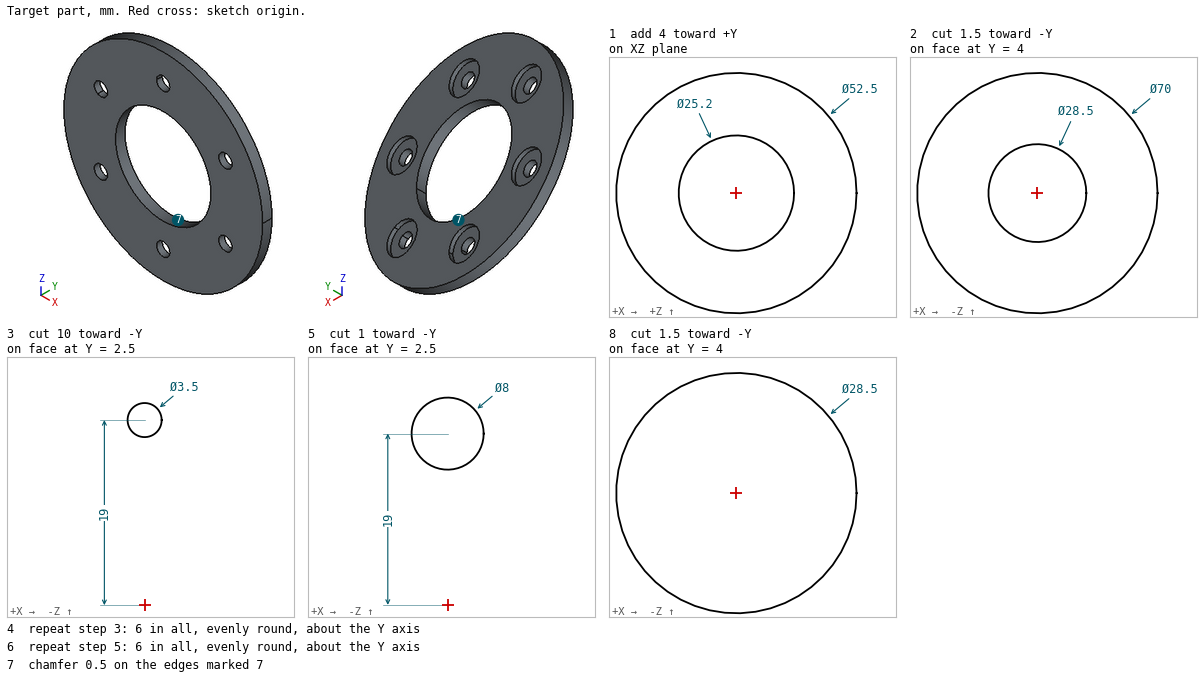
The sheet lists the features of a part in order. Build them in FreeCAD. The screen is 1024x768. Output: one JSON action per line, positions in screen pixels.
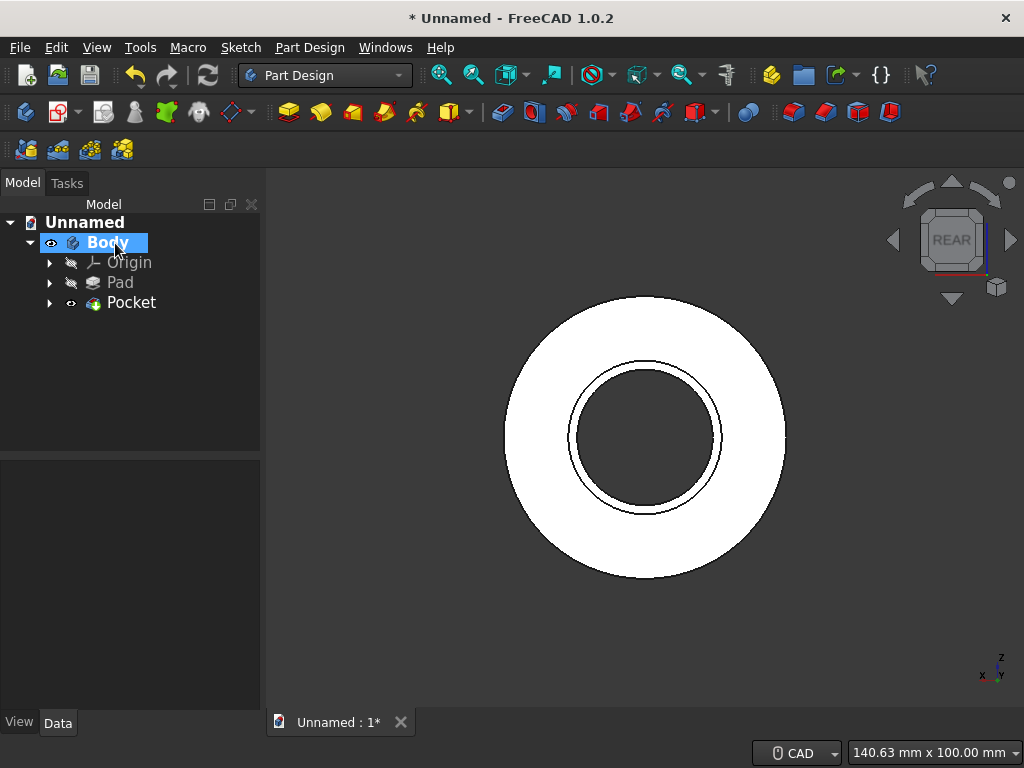
{"action": "left_click", "coordinate": [564, 356]}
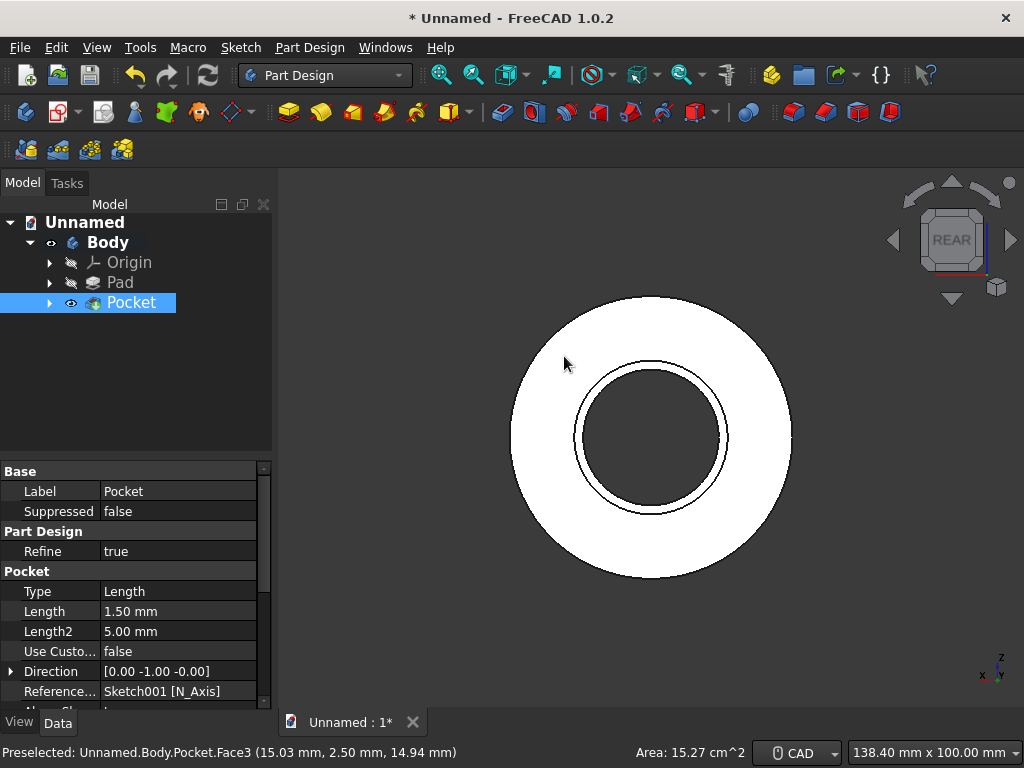
{"action": "left_click", "coordinate": [58, 112]}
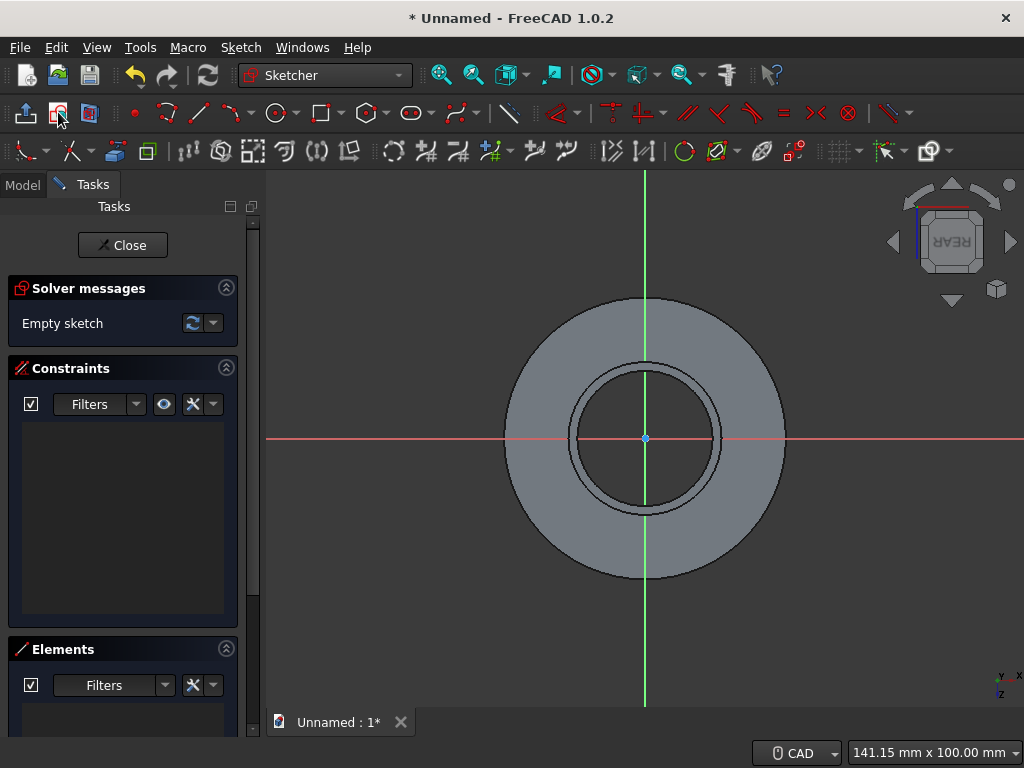
{"action": "left_click", "coordinate": [90, 114]}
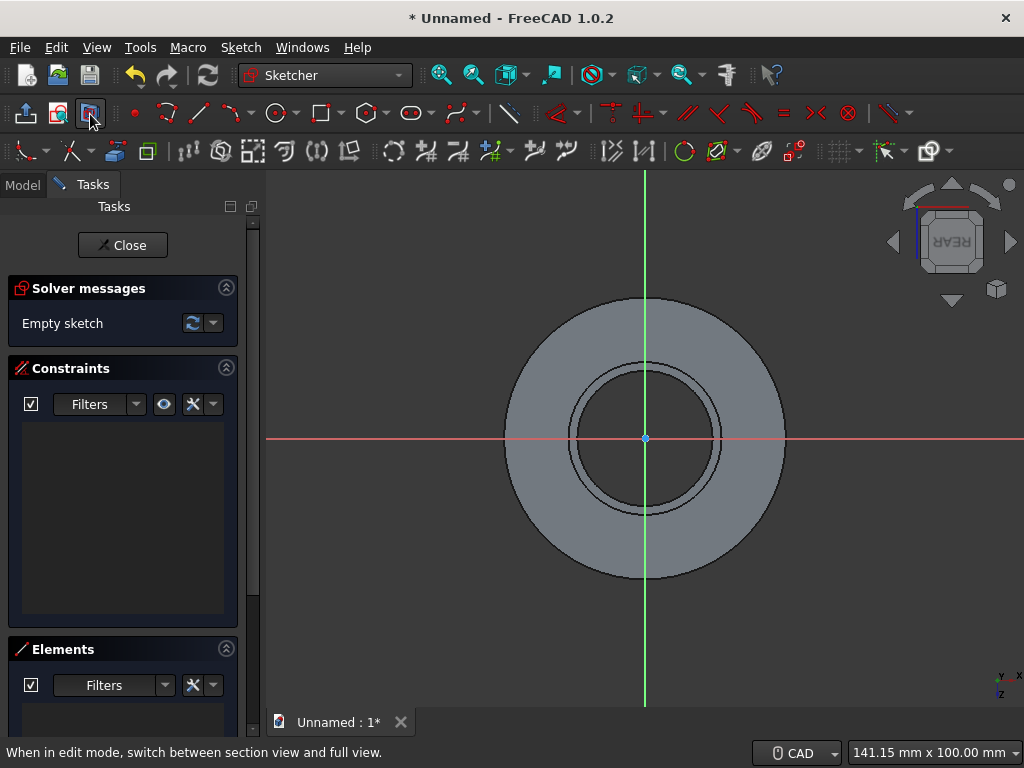
{"action": "scroll", "coordinate": [649, 330], "scroll_direction": "up", "scroll_amount": 14}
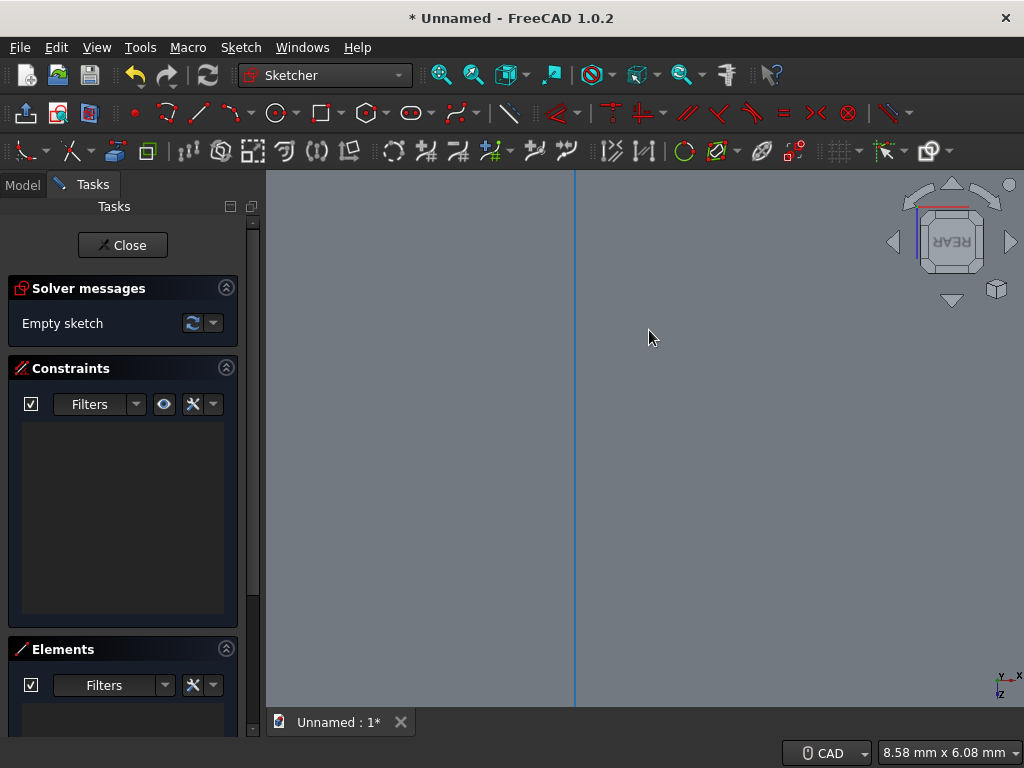
{"action": "left_click", "coordinate": [276, 114]}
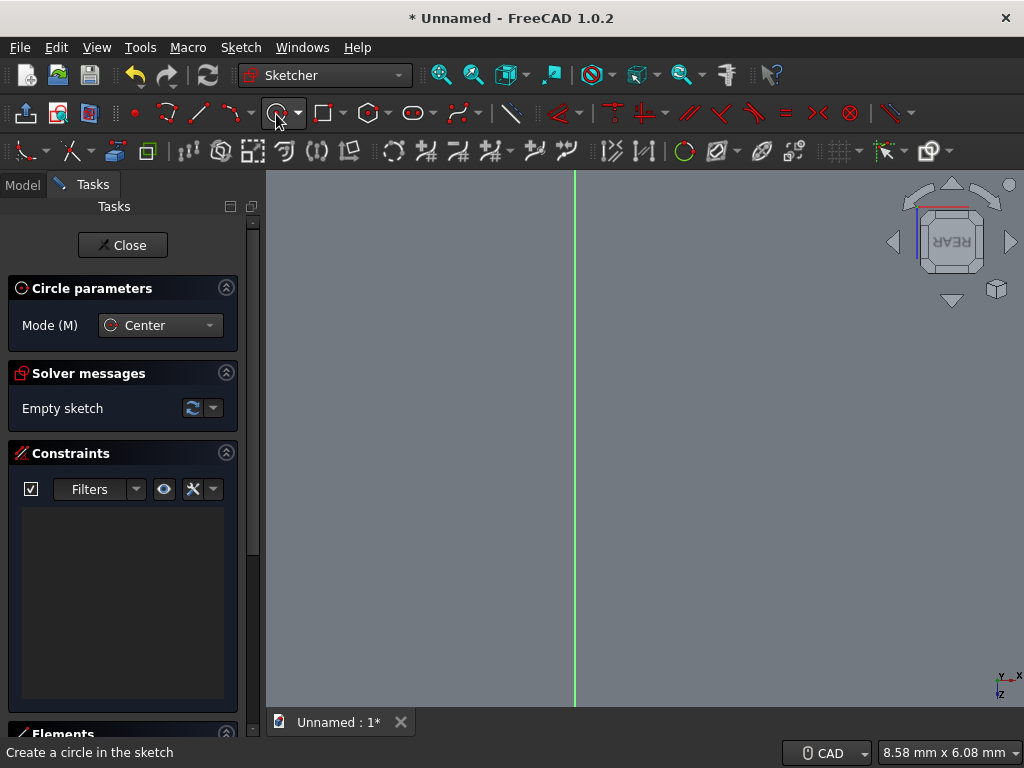
{"action": "left_click", "coordinate": [575, 432]}
{"action": "mouse_move", "coordinate": [685, 323]}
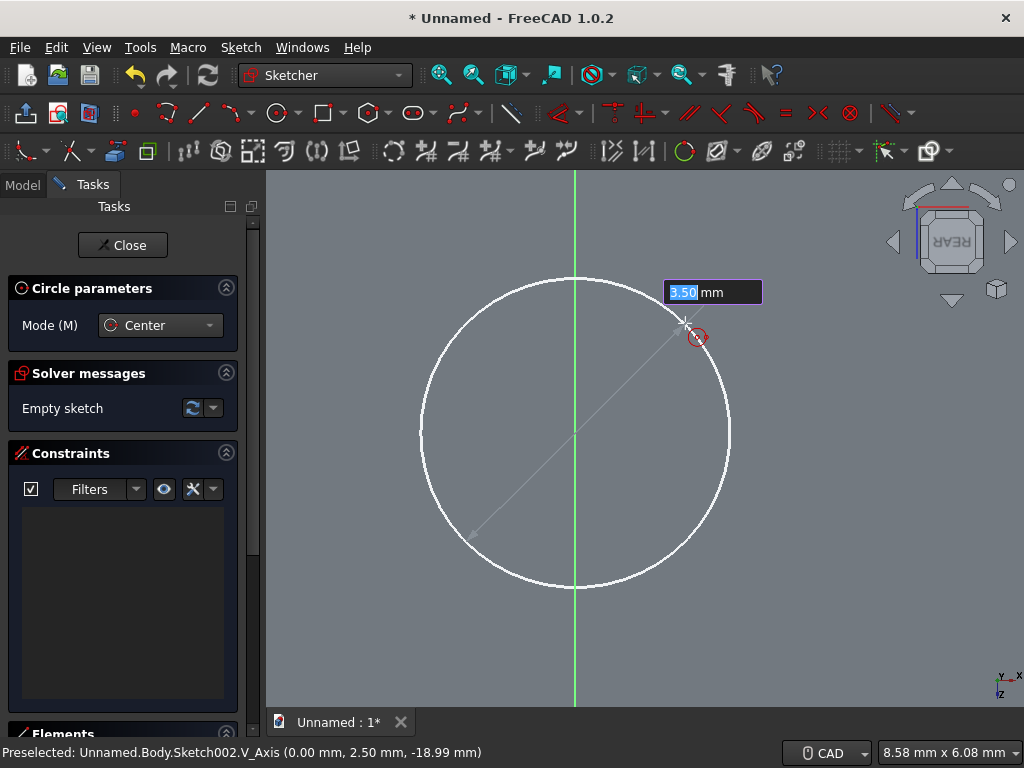
{"action": "type", "text": "3.5"}
{"action": "key", "text": "Return"}
{"action": "key", "text": "Escape"}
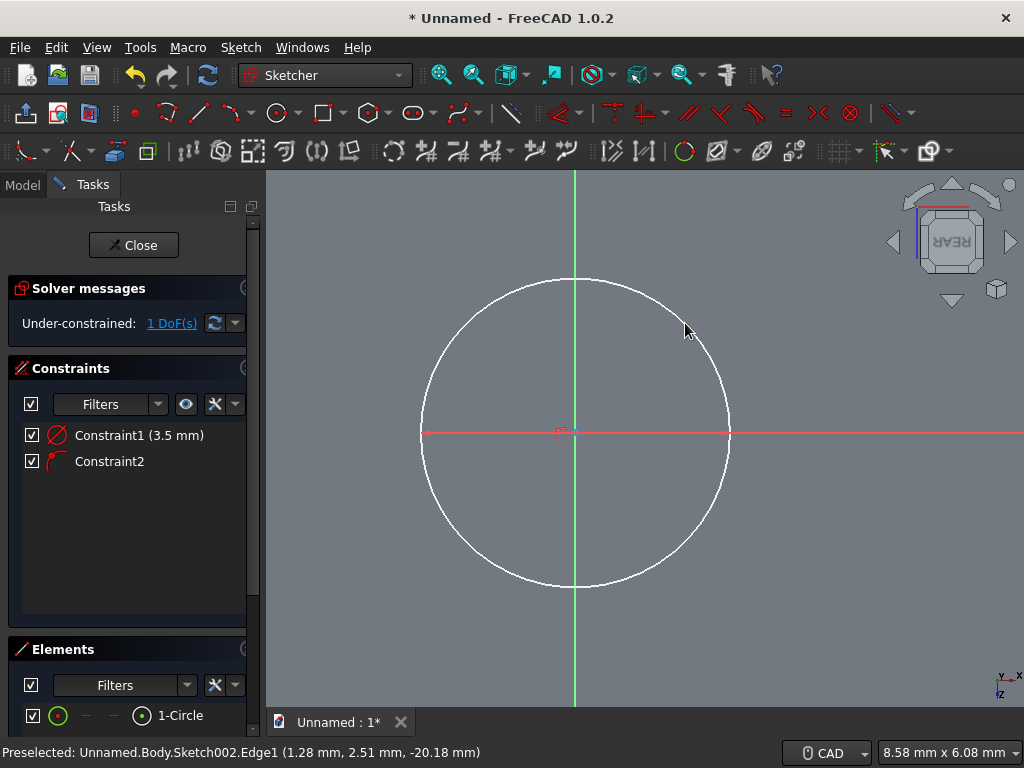
{"action": "left_click", "coordinate": [558, 114]}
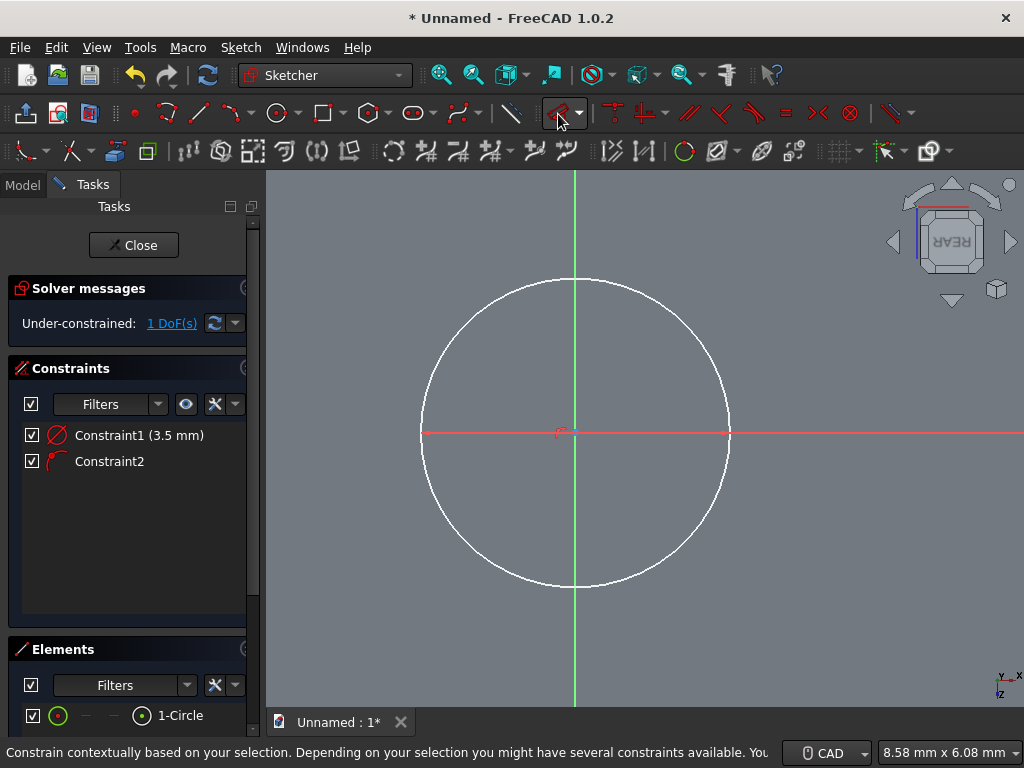
{"action": "left_click", "coordinate": [575, 433]}
{"action": "left_click", "coordinate": [609, 556]}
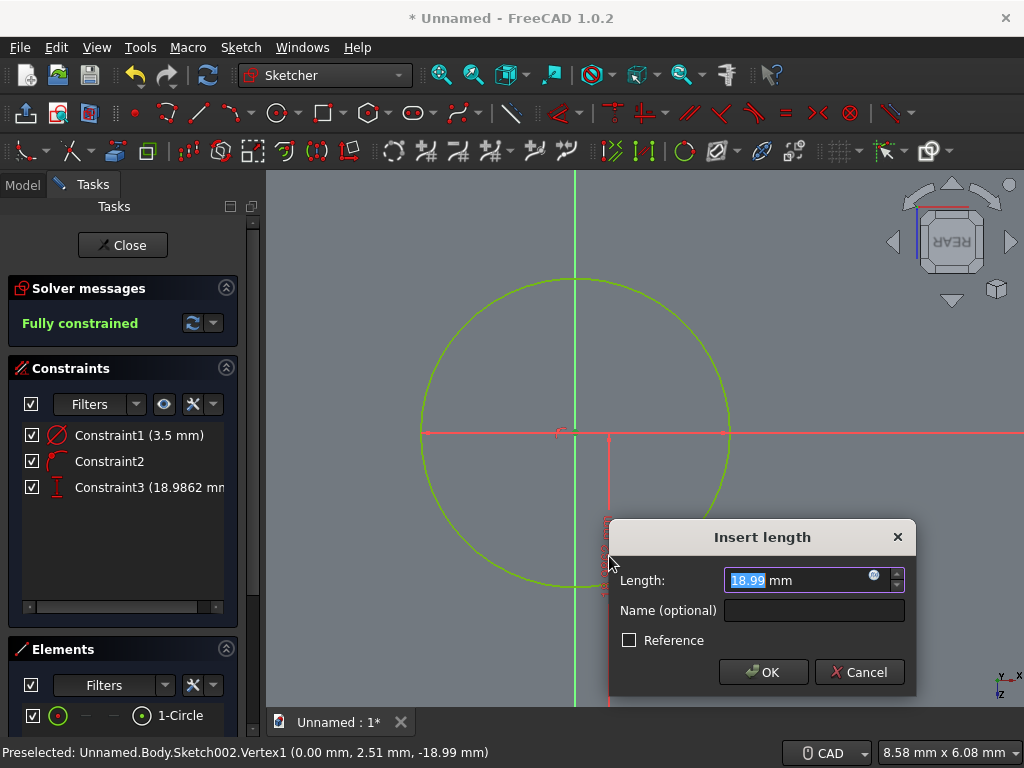
{"action": "type", "text": "19"}
{"action": "key", "text": "Return"}
{"action": "key", "text": "Escape"}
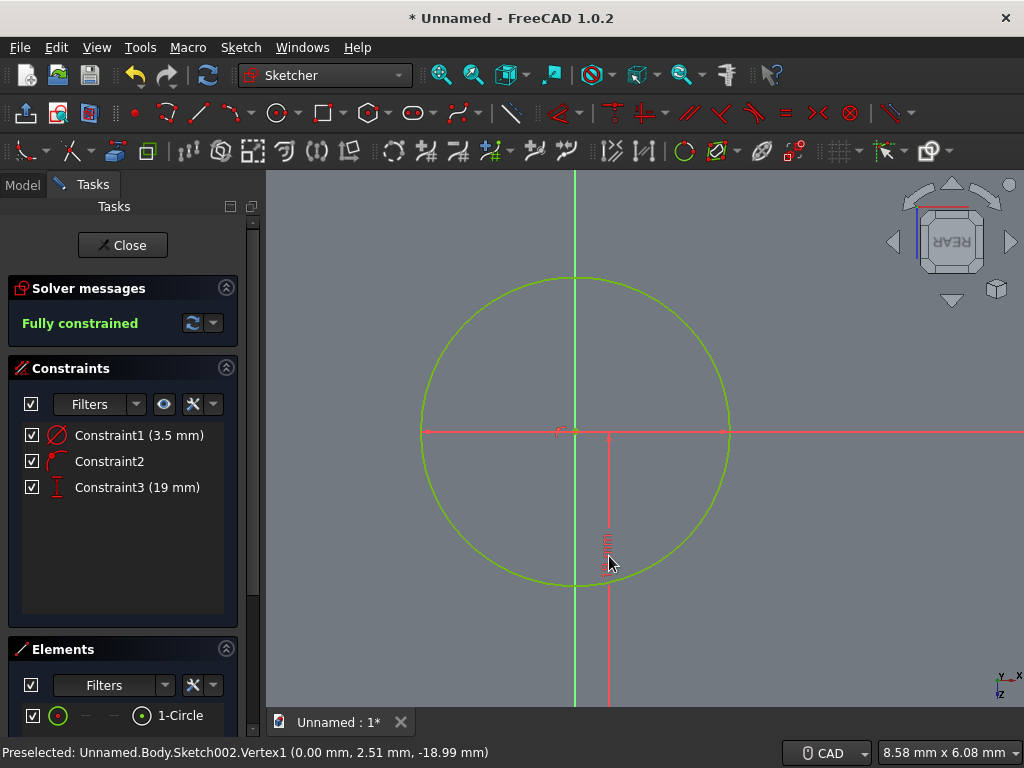
{"action": "left_click", "coordinate": [123, 245]}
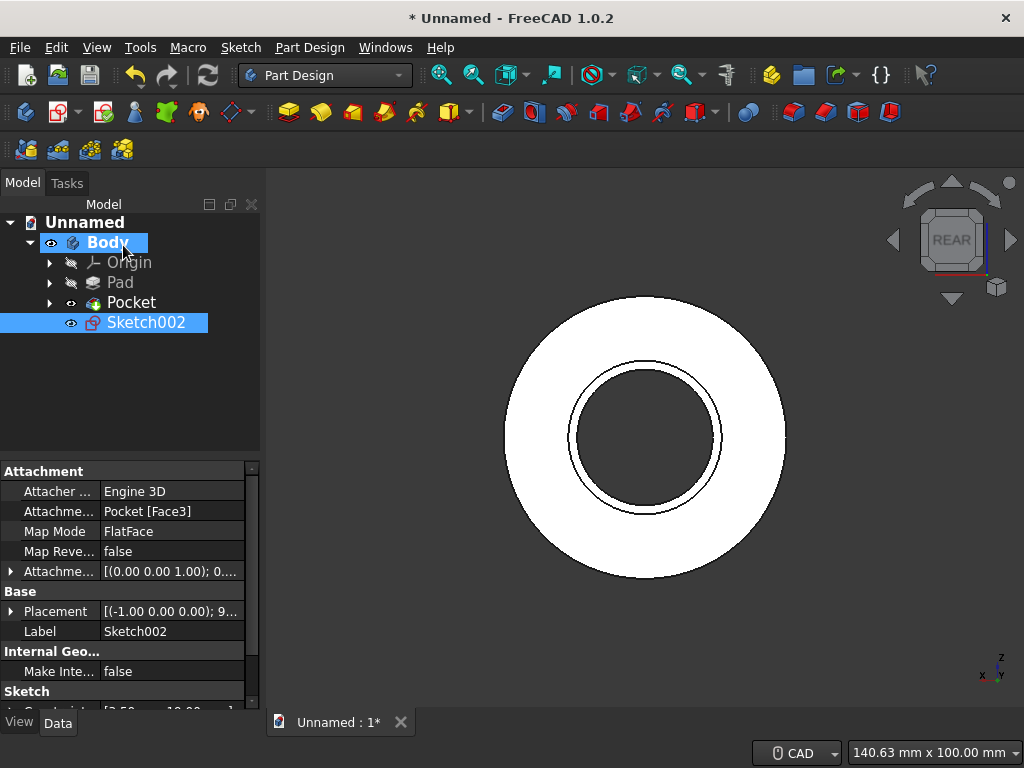
{"action": "left_click", "coordinate": [504, 112]}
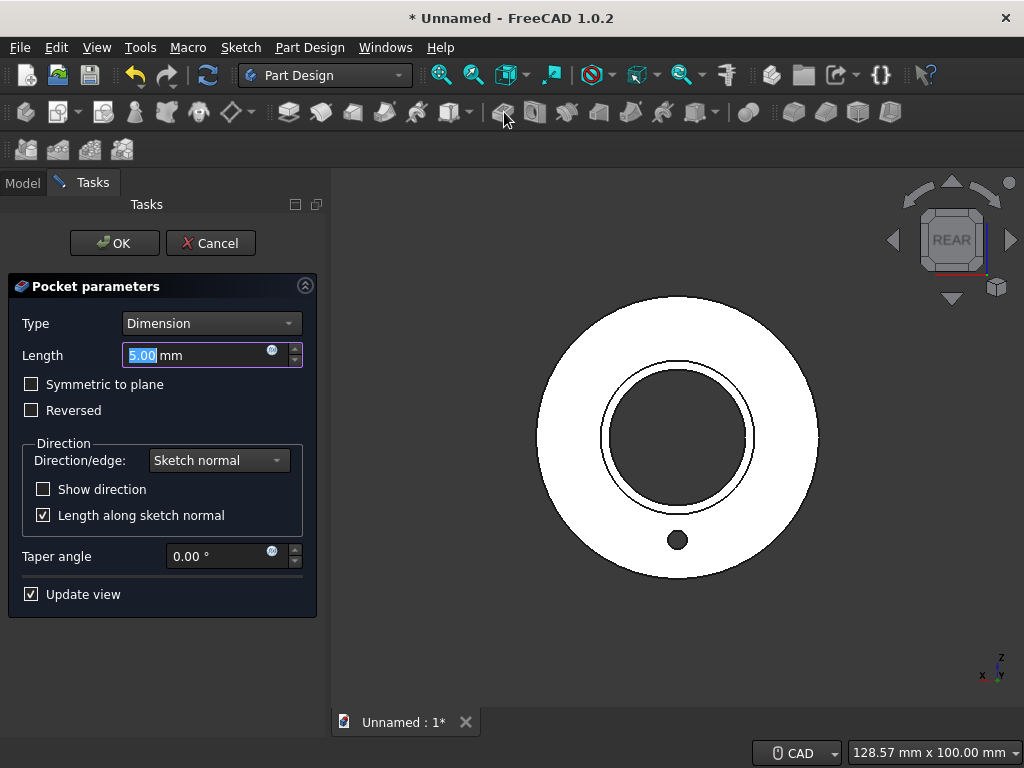
{"action": "type", "text": "10"}
{"action": "key", "text": "Tab"}